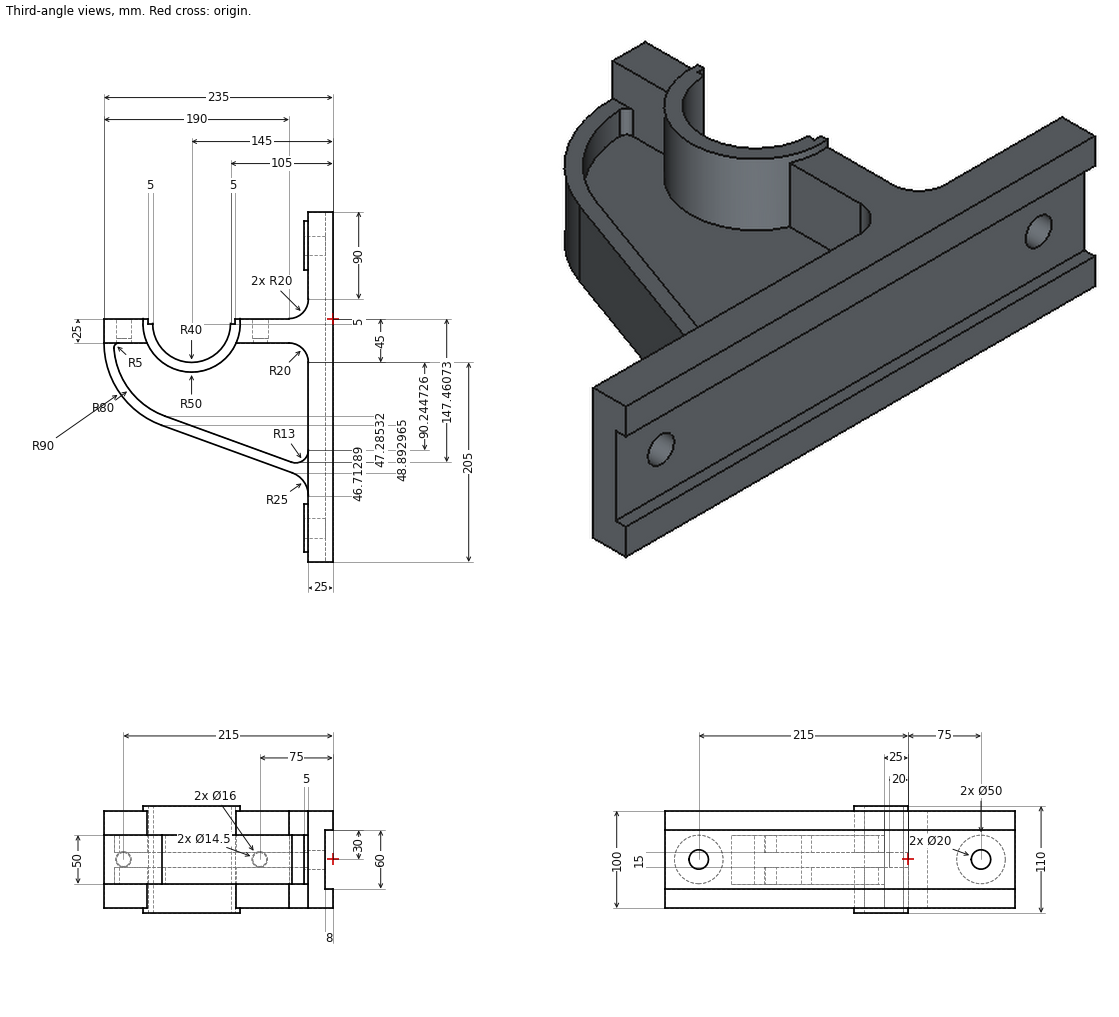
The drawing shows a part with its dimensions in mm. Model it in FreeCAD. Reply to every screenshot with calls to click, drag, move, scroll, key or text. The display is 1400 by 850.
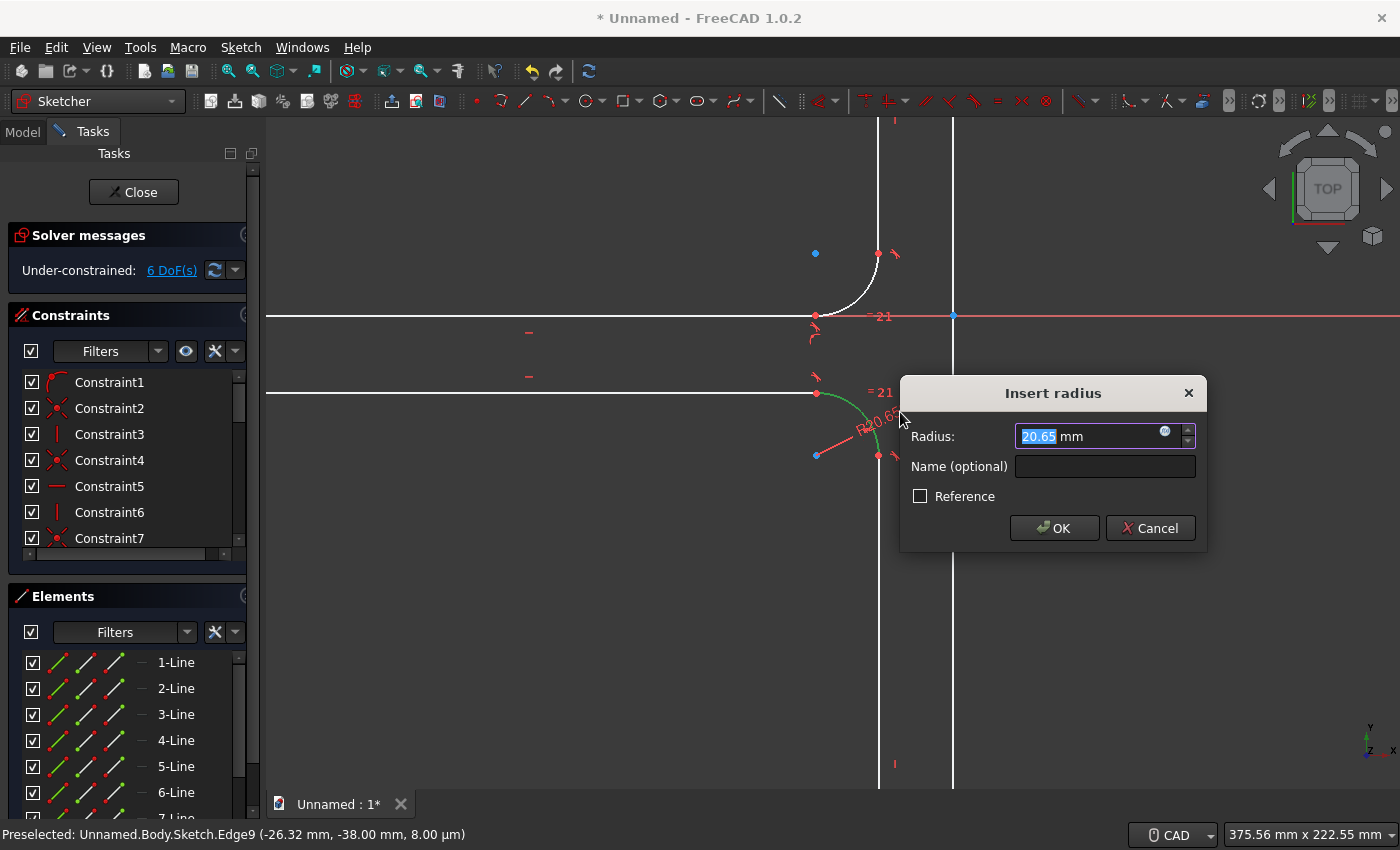
text(20)
key(Return)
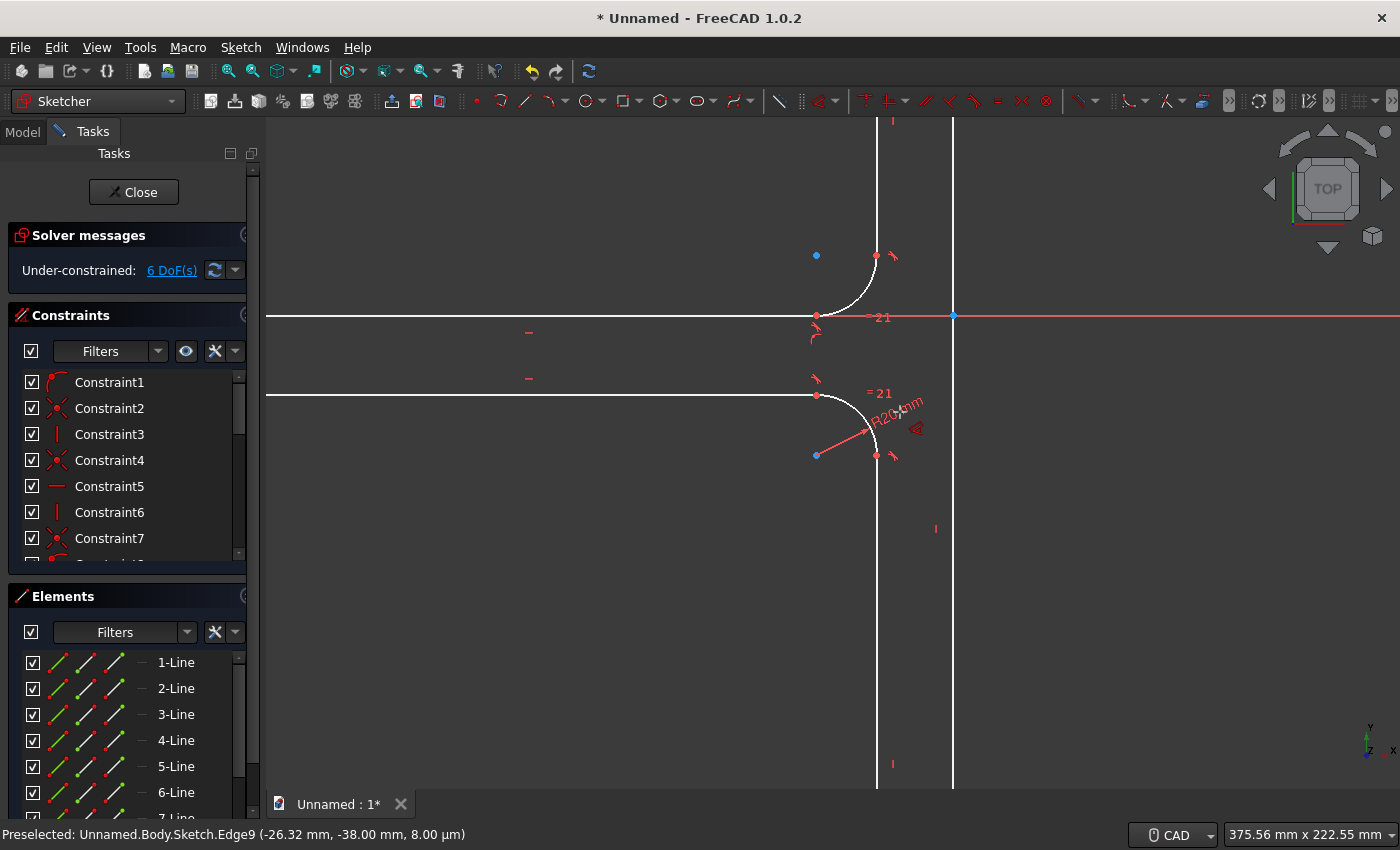
scroll(861, 410, down, 5)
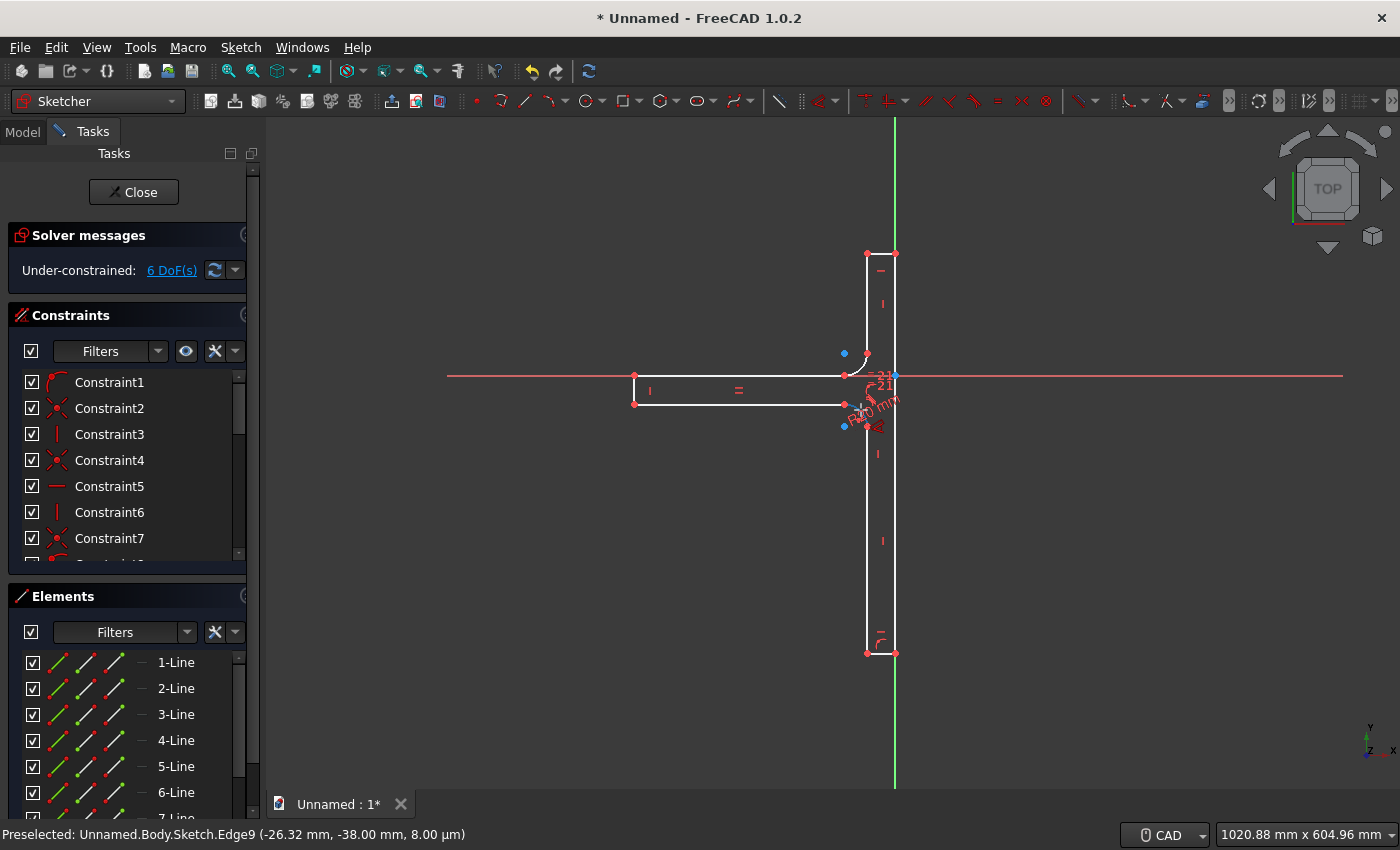
scroll(634, 384, up, 3)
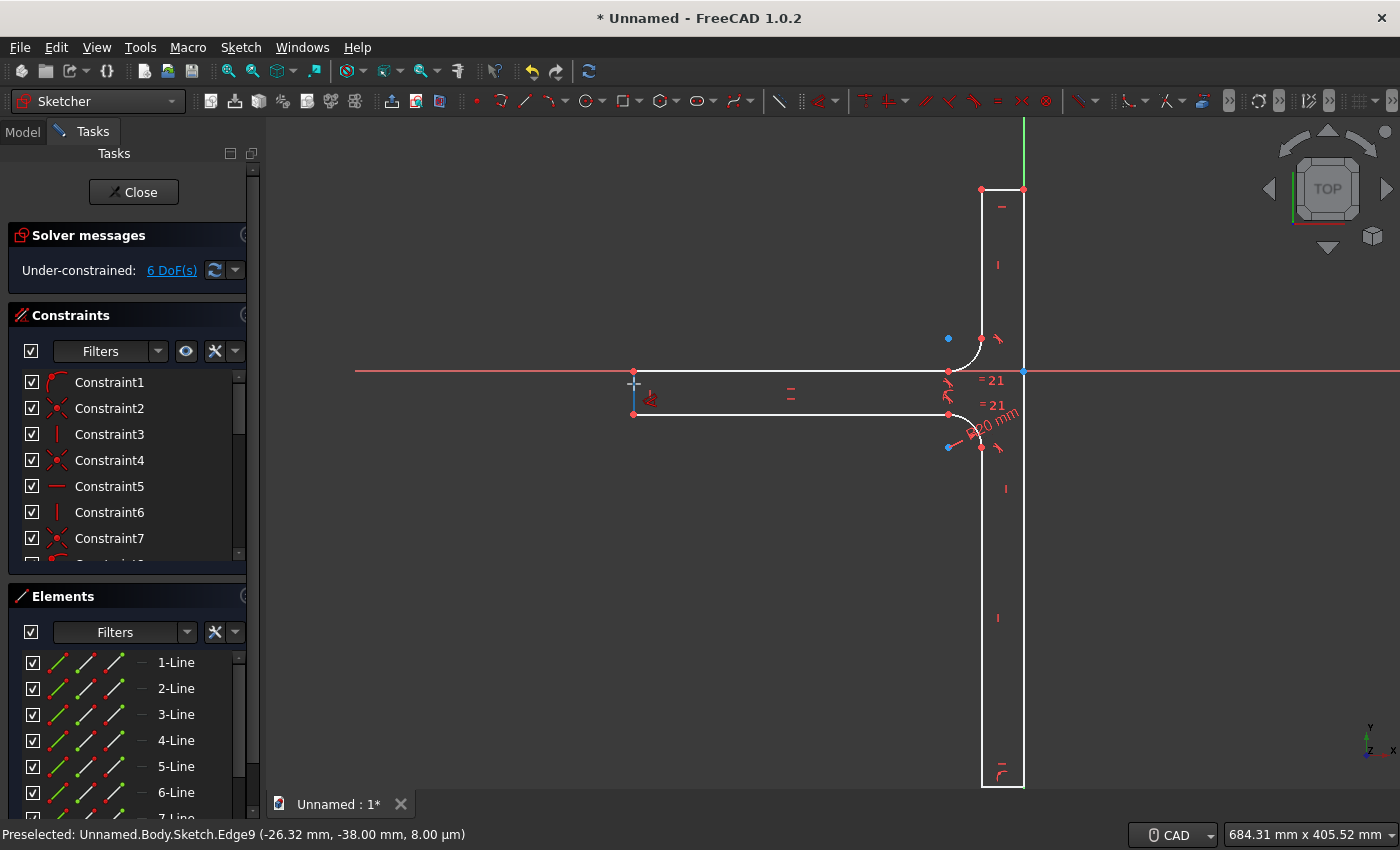
click(634, 384)
click(600, 395)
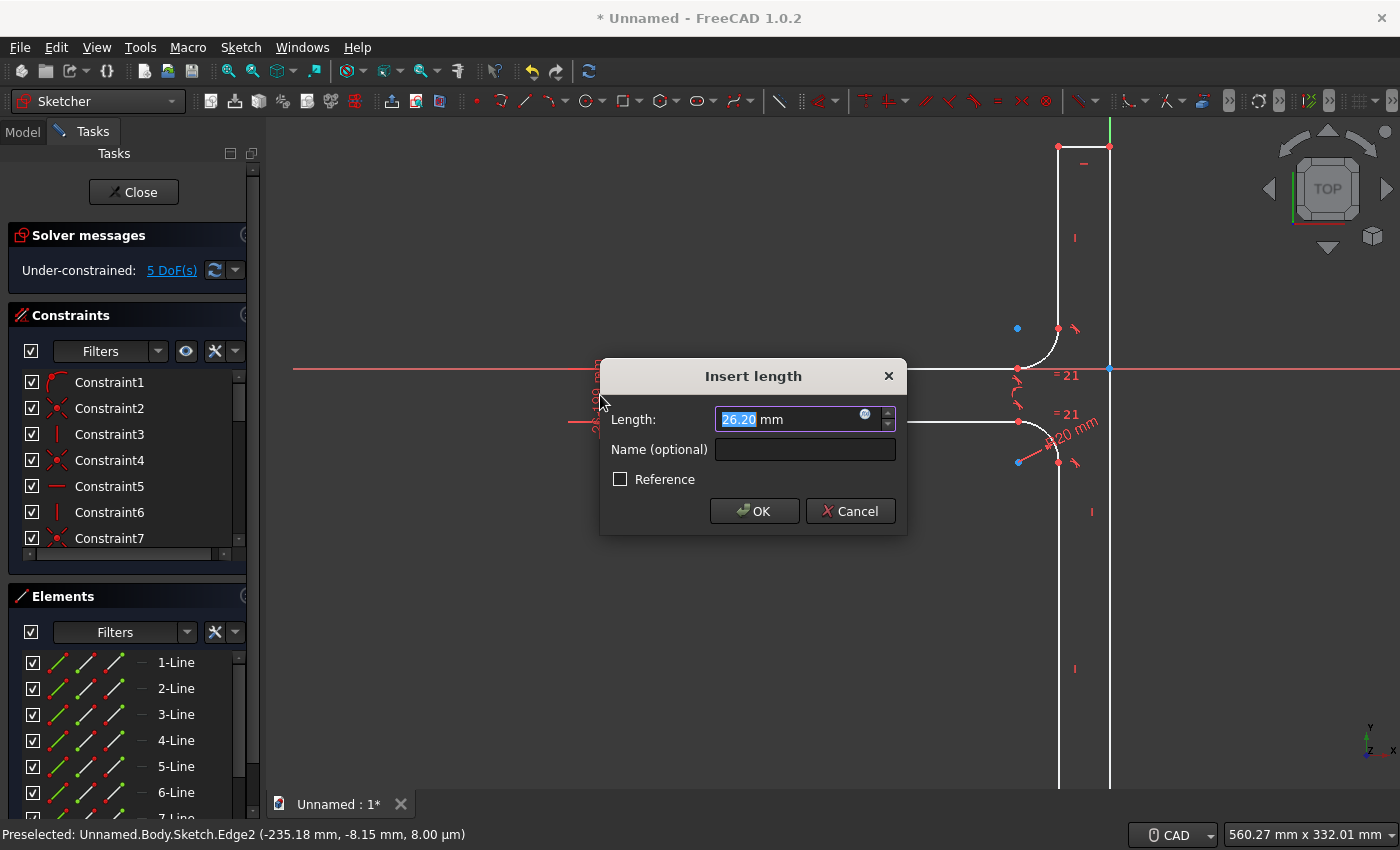
text(25)
key(Return)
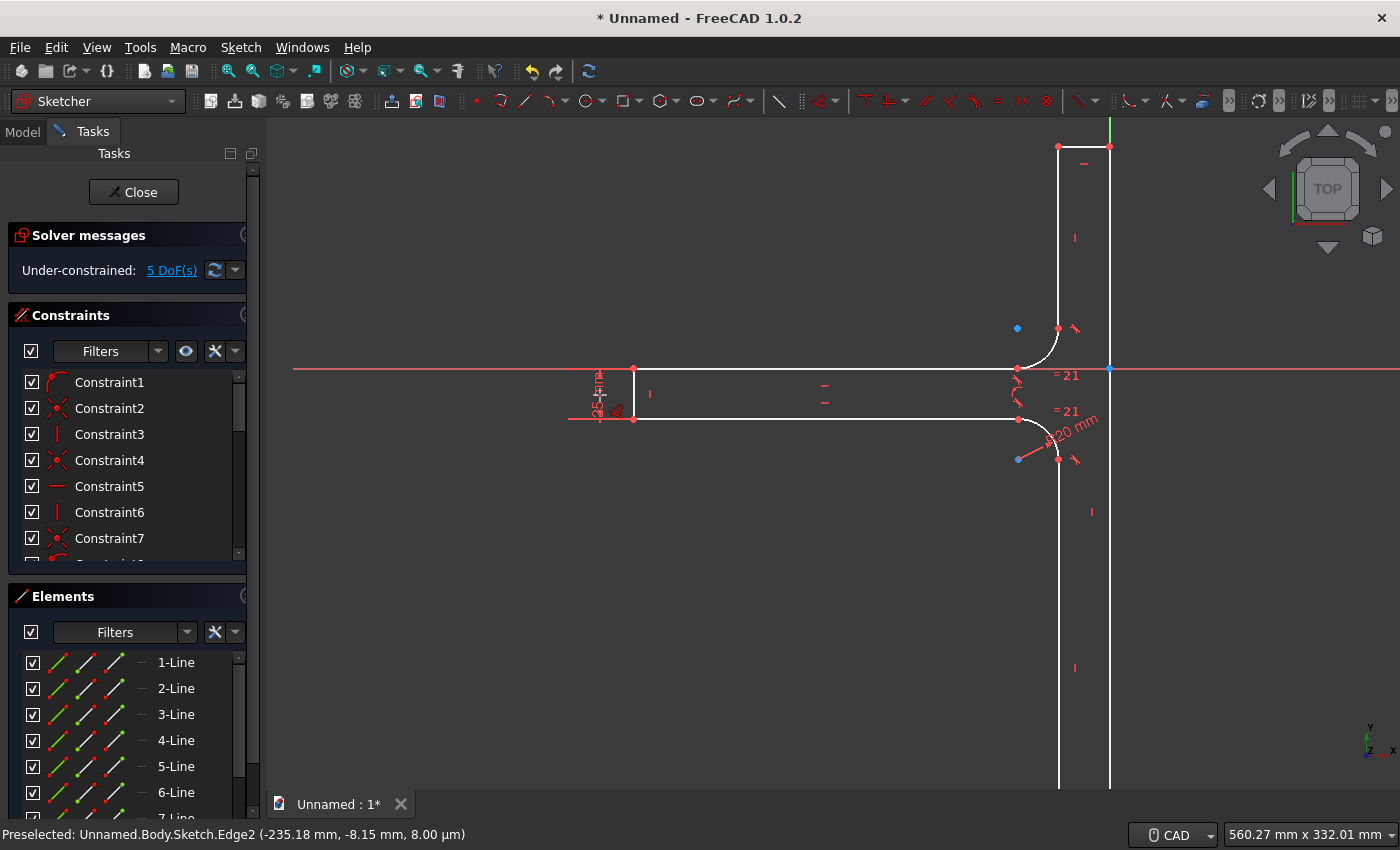
scroll(634, 383, down, 3)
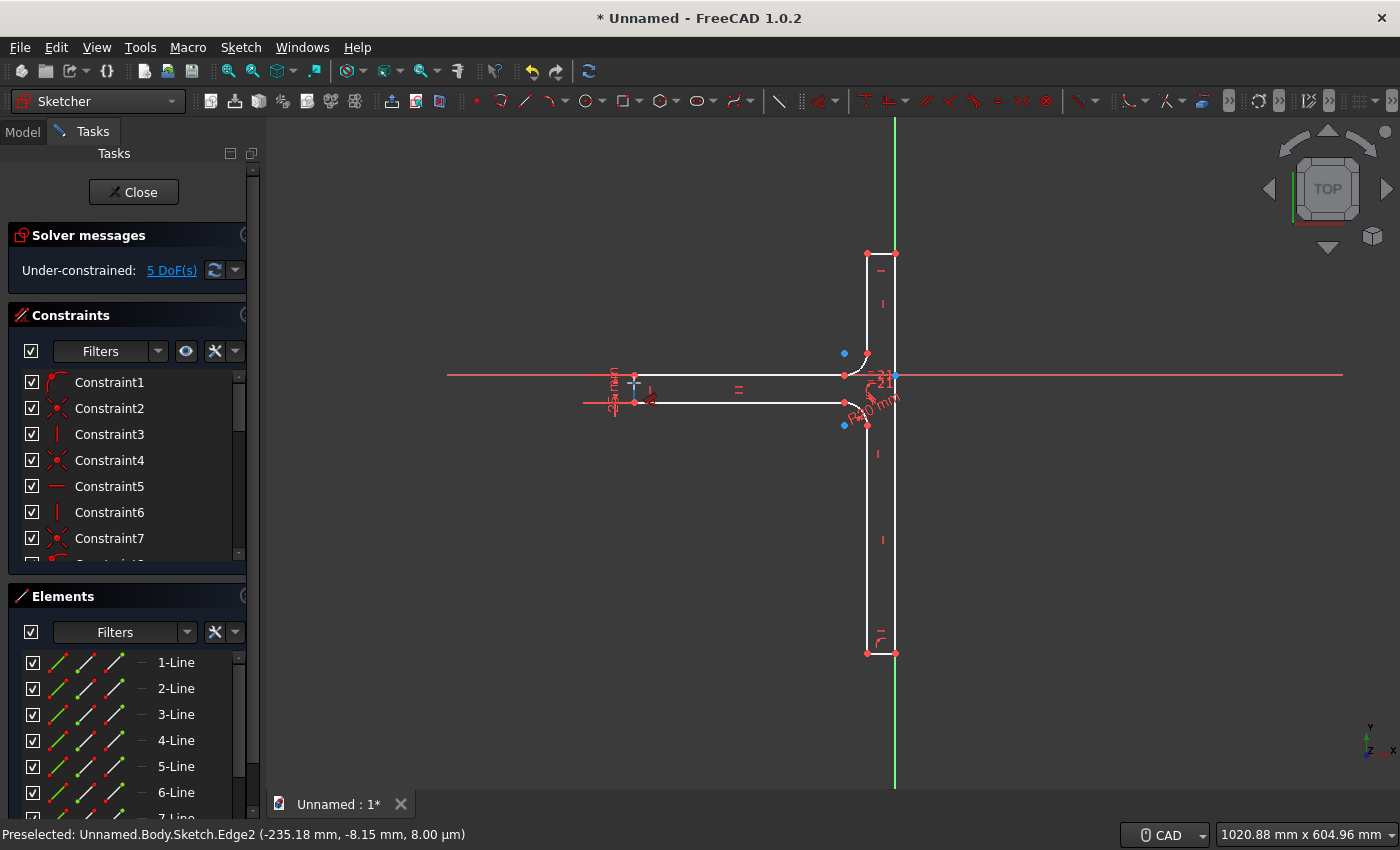
scroll(876, 654, up, 3)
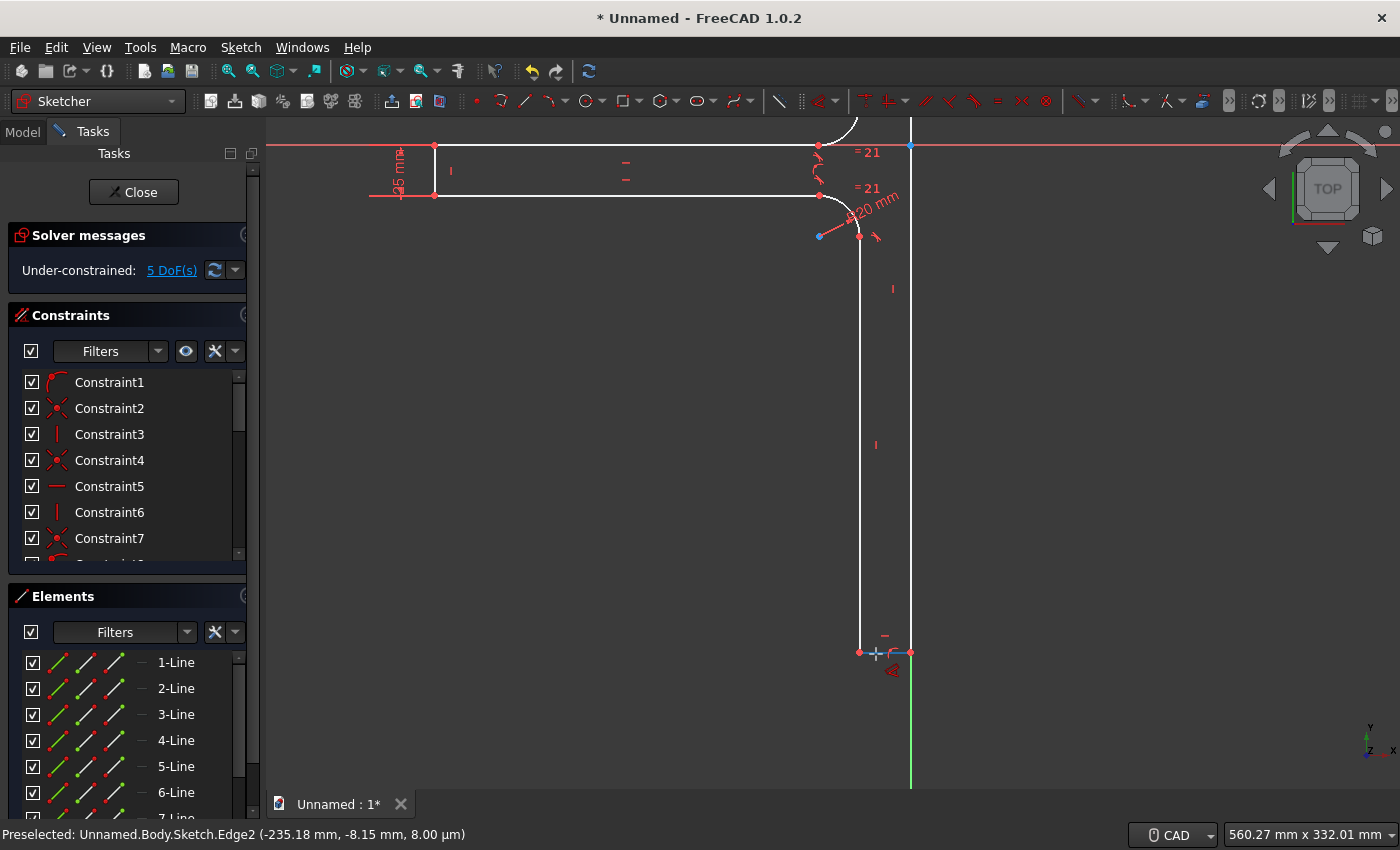
click(875, 653)
click(885, 687)